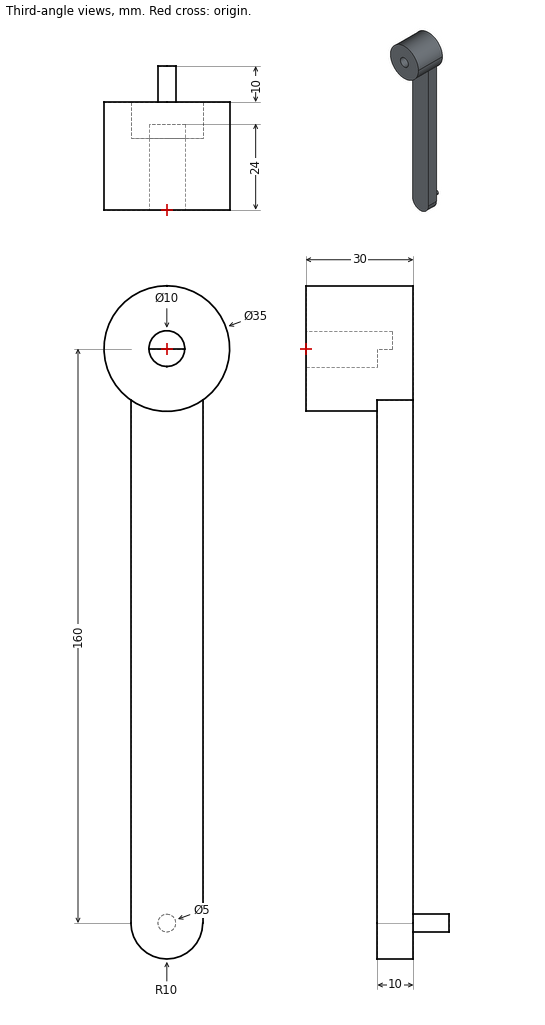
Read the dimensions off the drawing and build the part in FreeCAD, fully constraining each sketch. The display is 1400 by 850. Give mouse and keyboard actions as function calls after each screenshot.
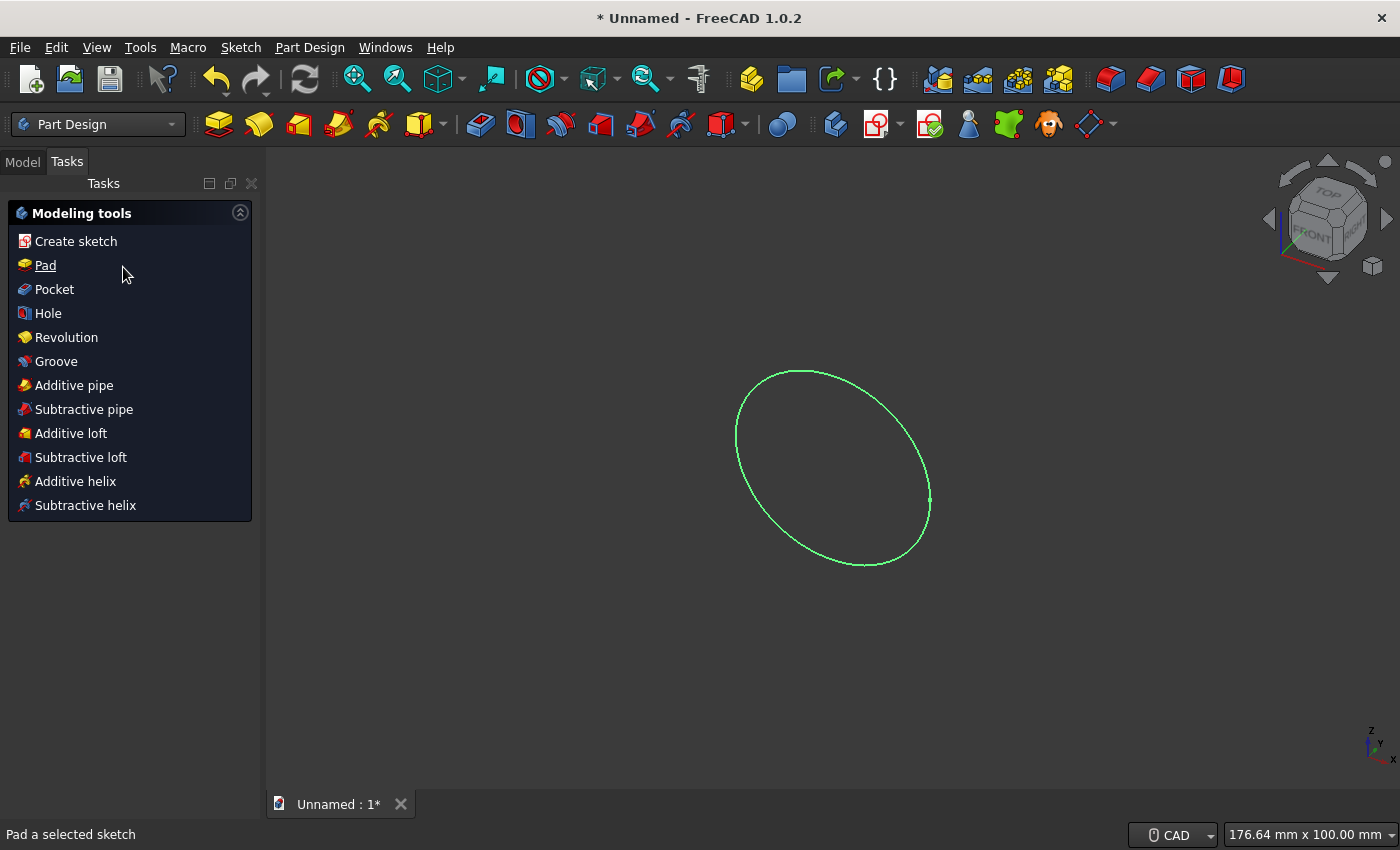
click(220, 124)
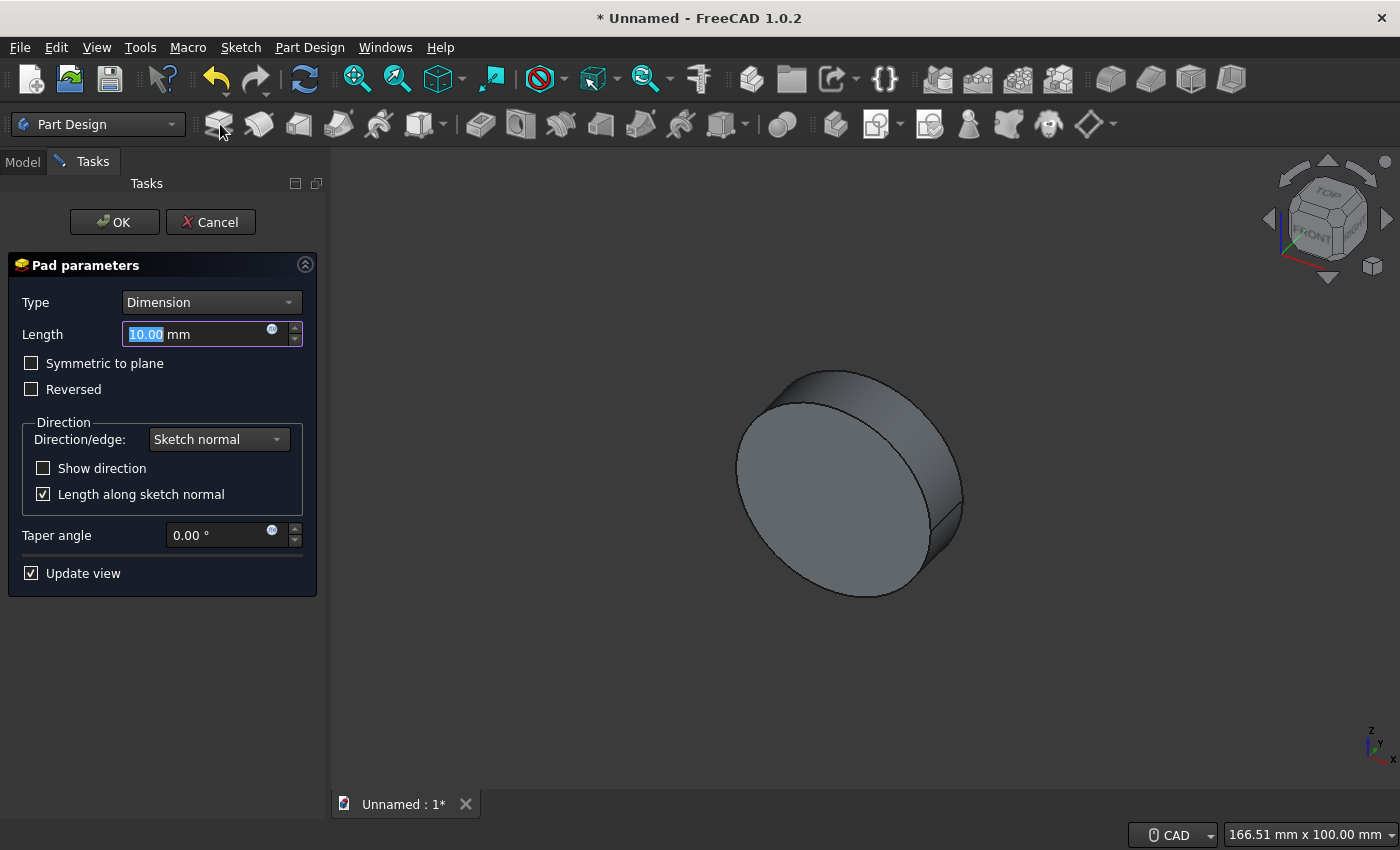
text(30)
key(Tab)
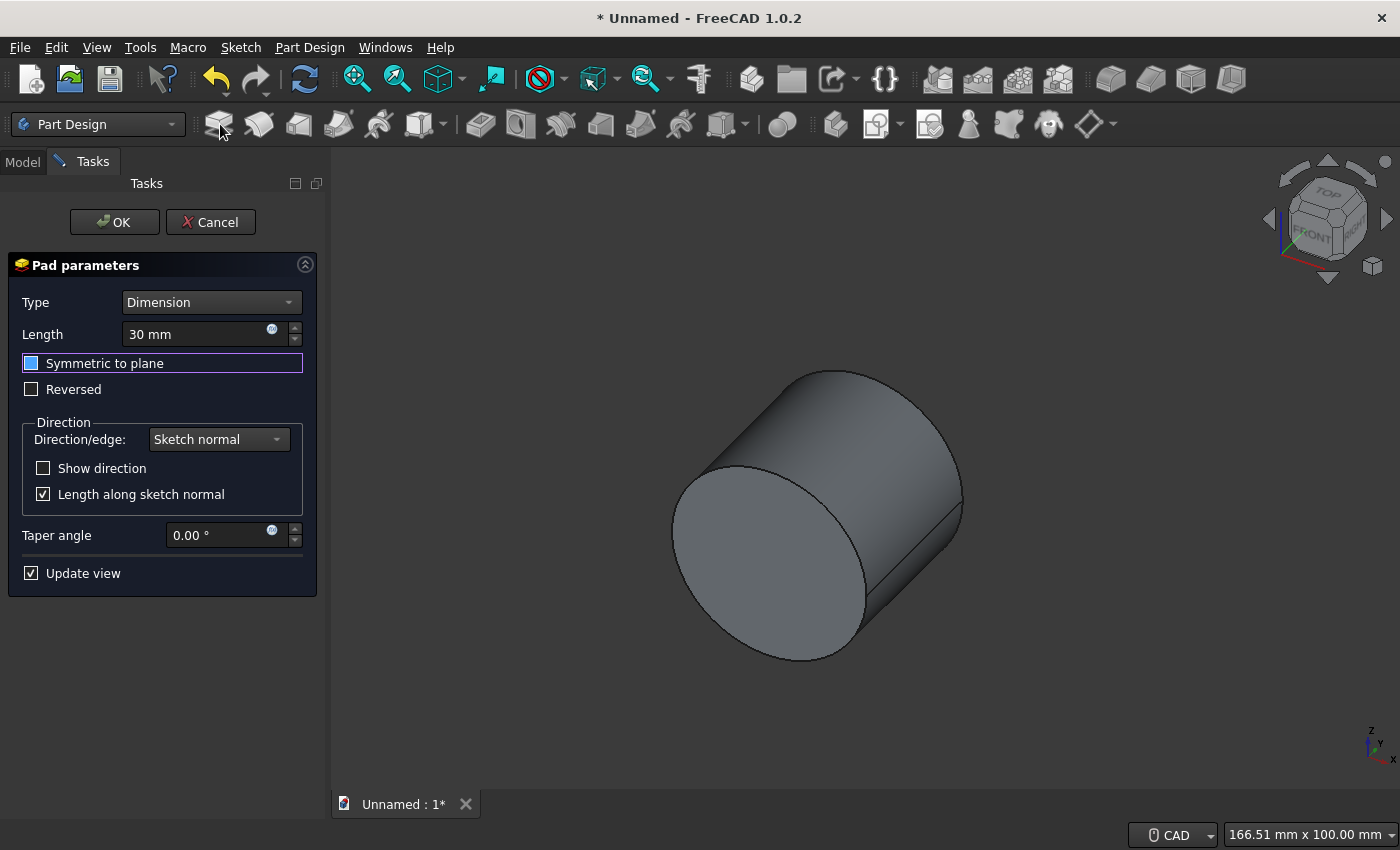
click(30, 389)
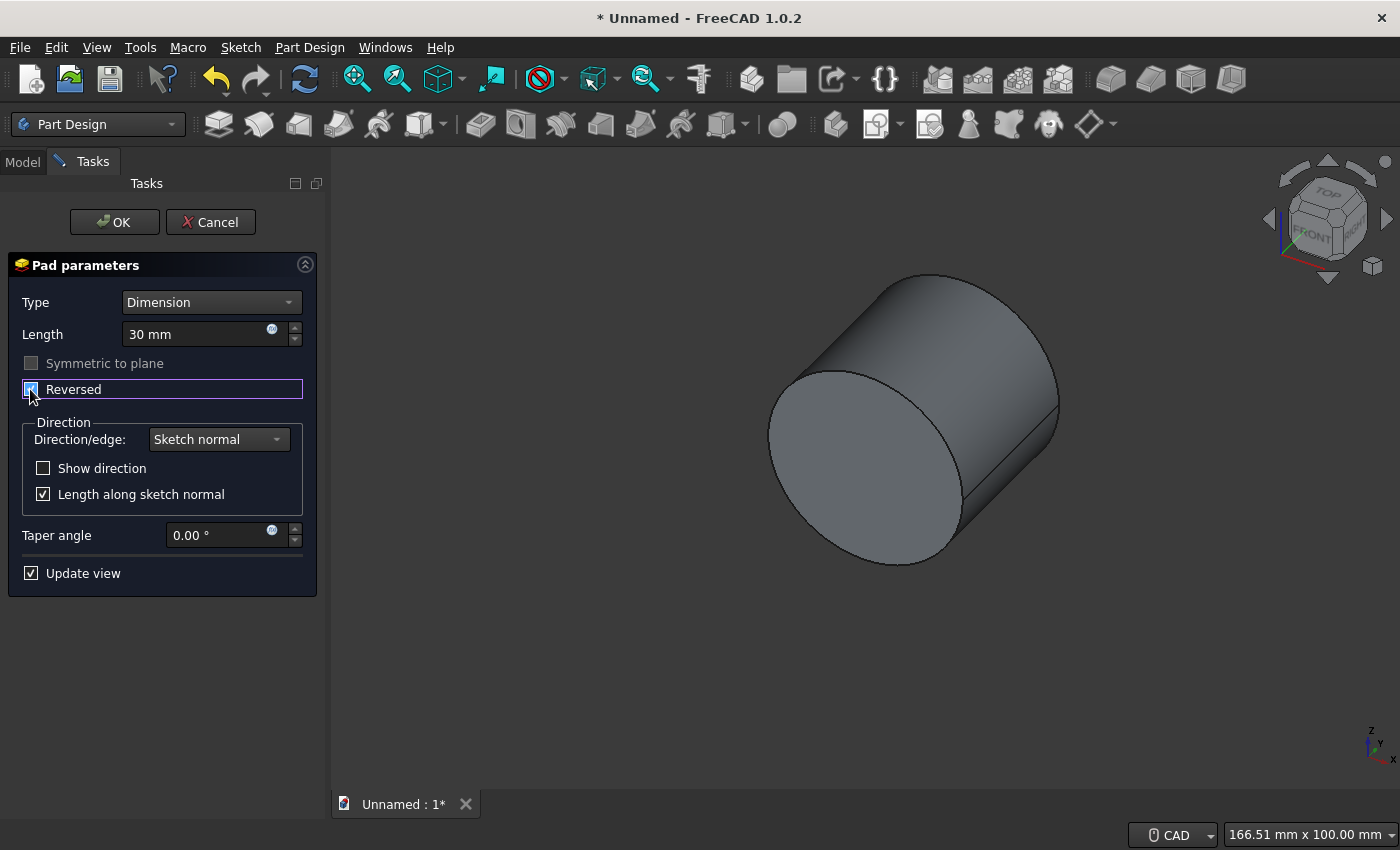
click(115, 222)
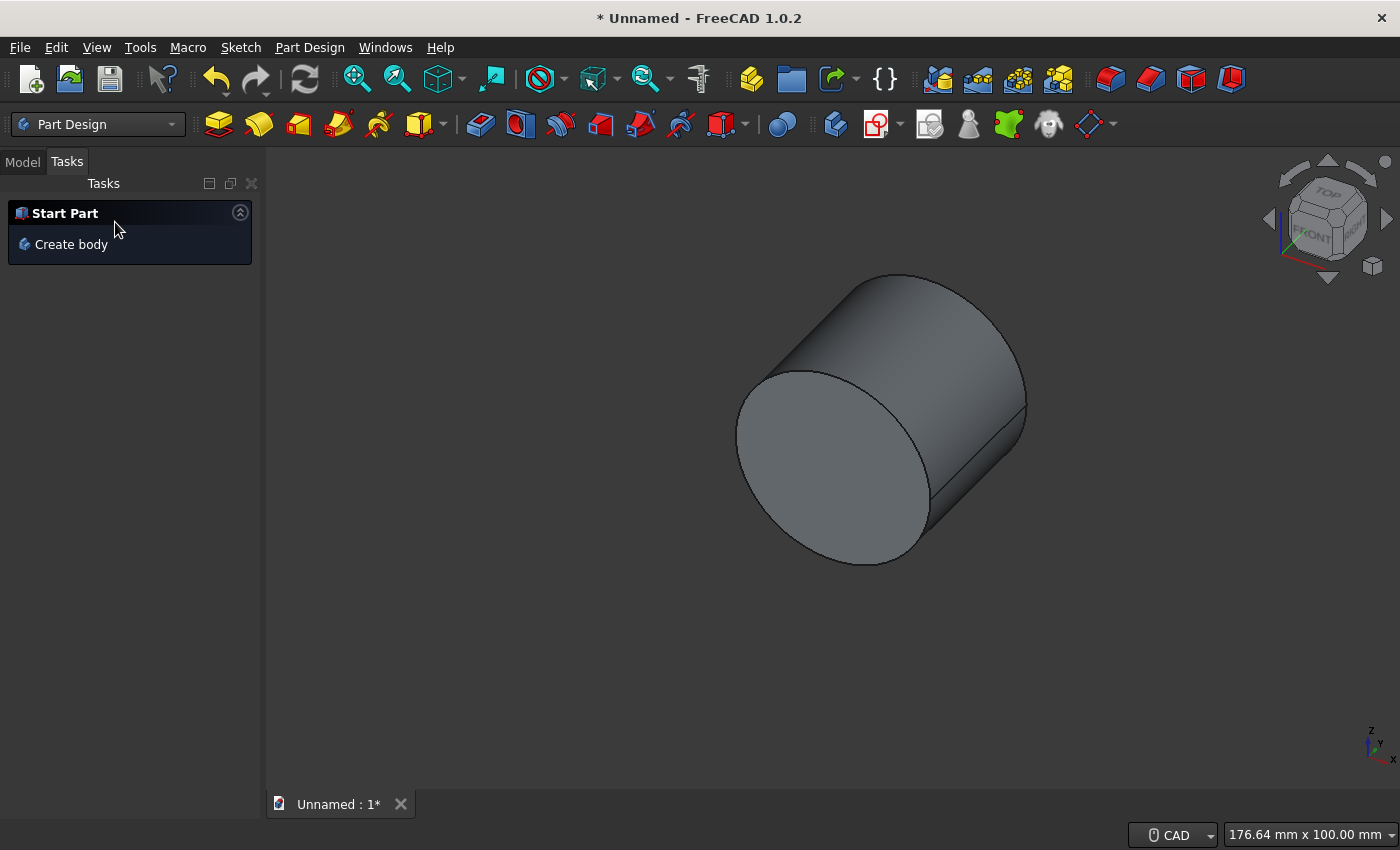
click(876, 124)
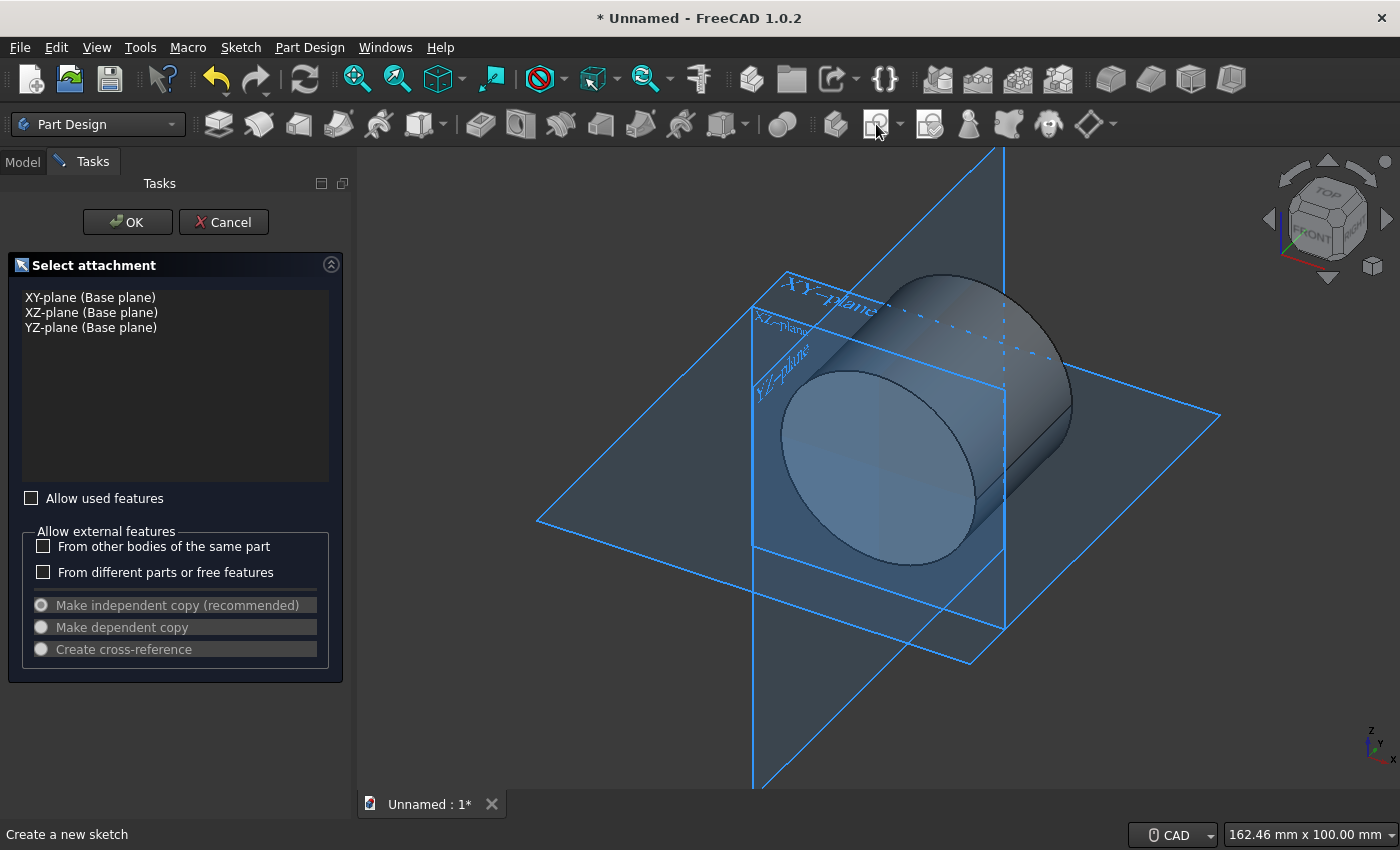
click(82, 312)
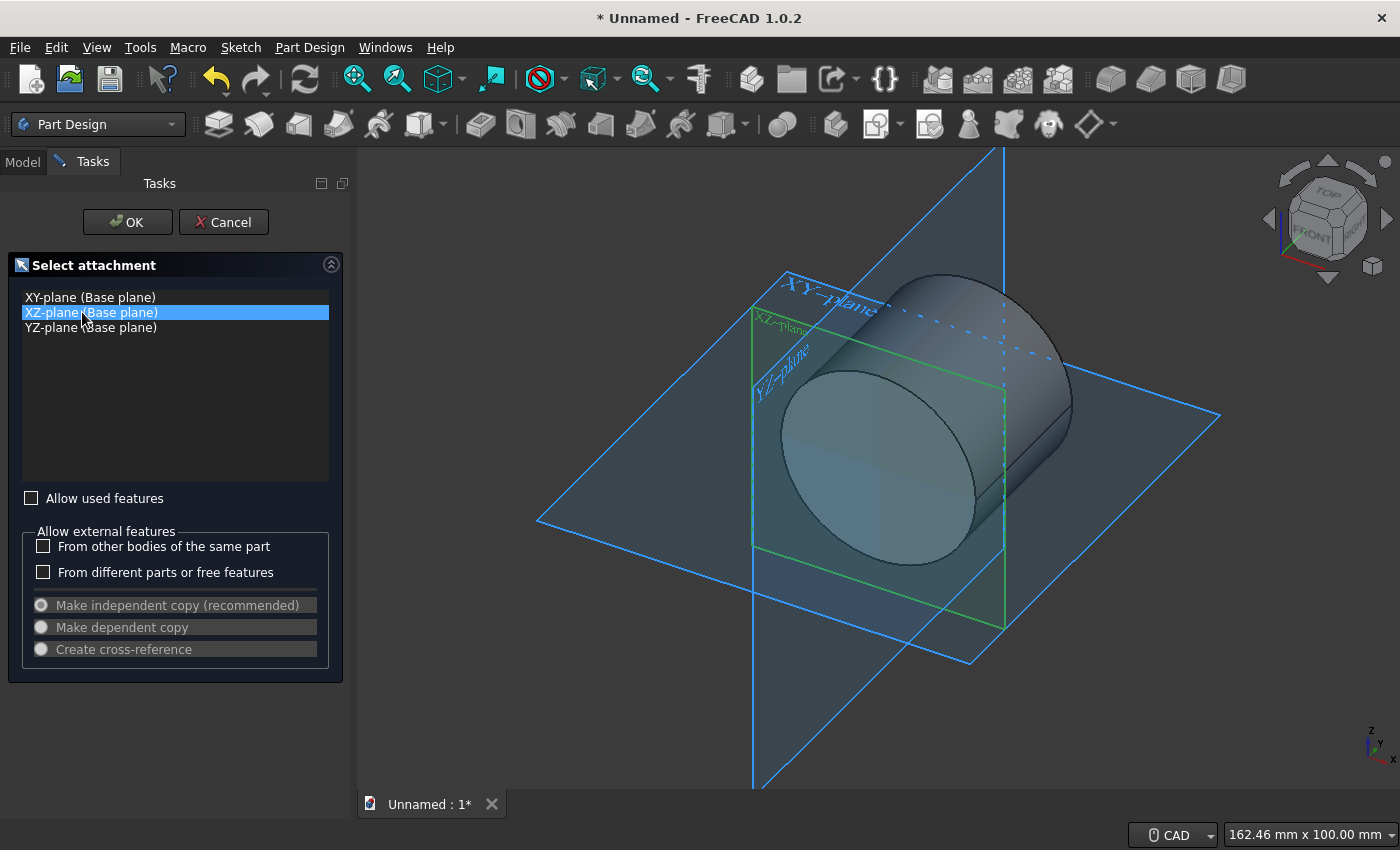
click(128, 222)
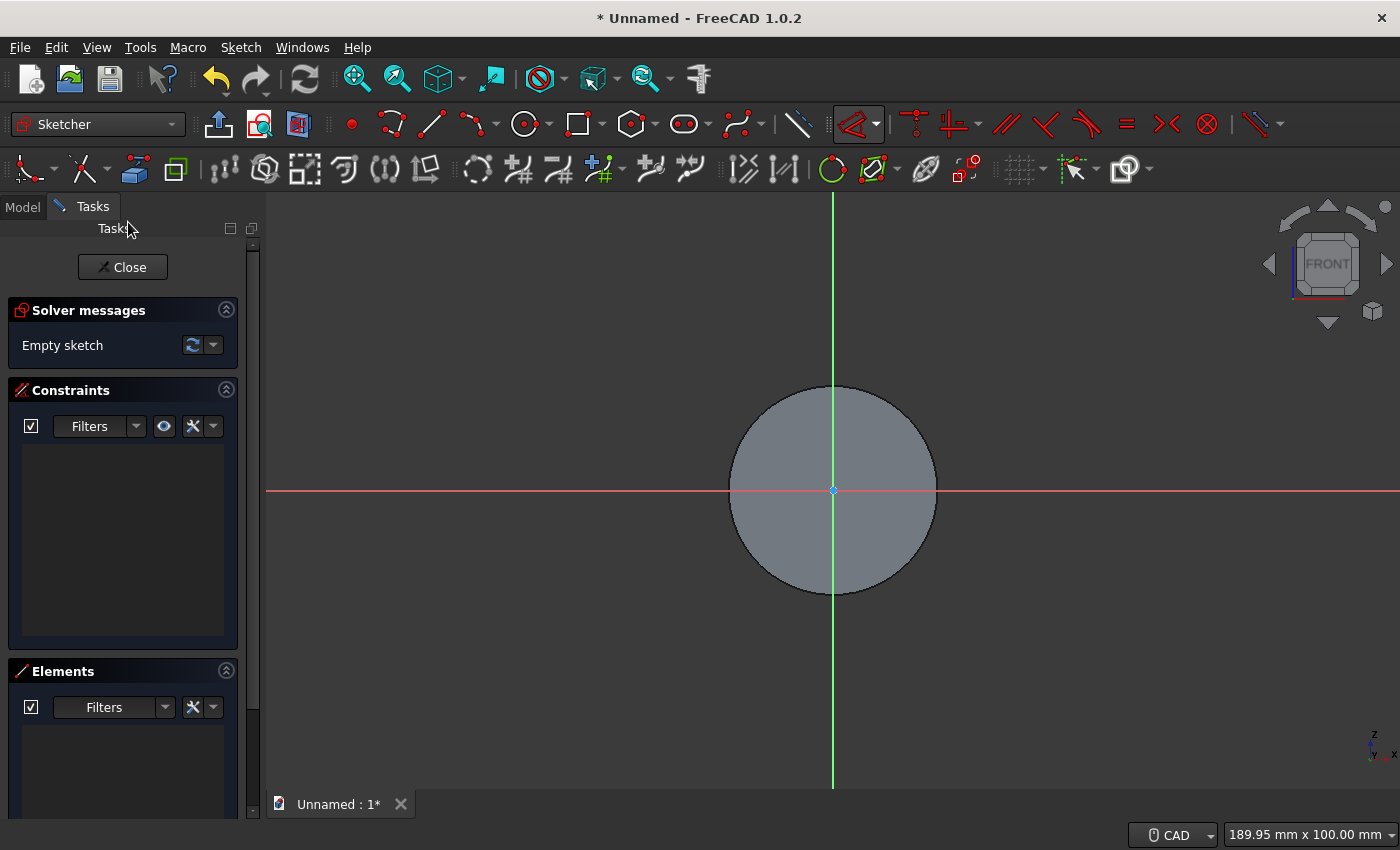
scroll(847, 490, up, 9)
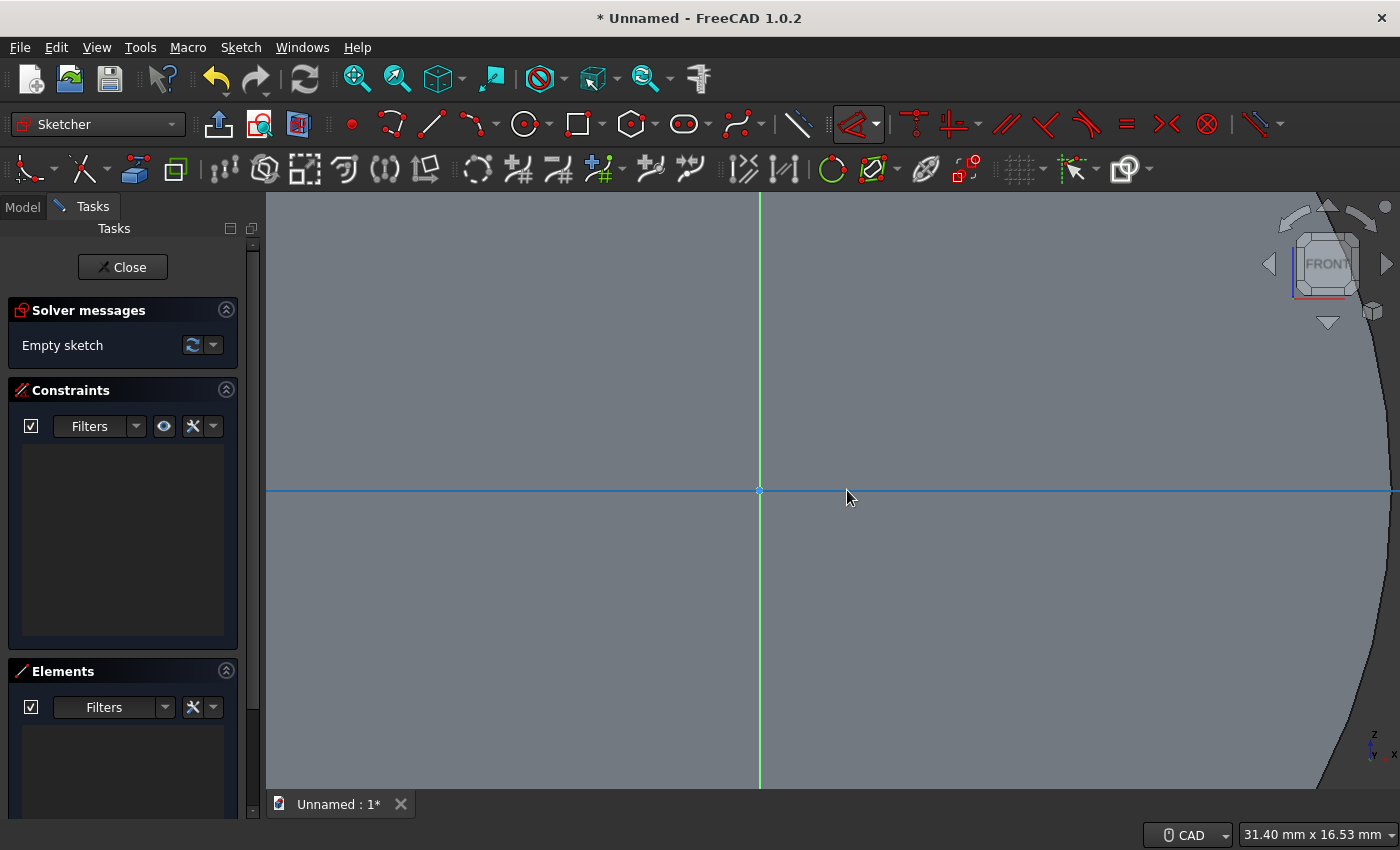
key(g)
key(c)